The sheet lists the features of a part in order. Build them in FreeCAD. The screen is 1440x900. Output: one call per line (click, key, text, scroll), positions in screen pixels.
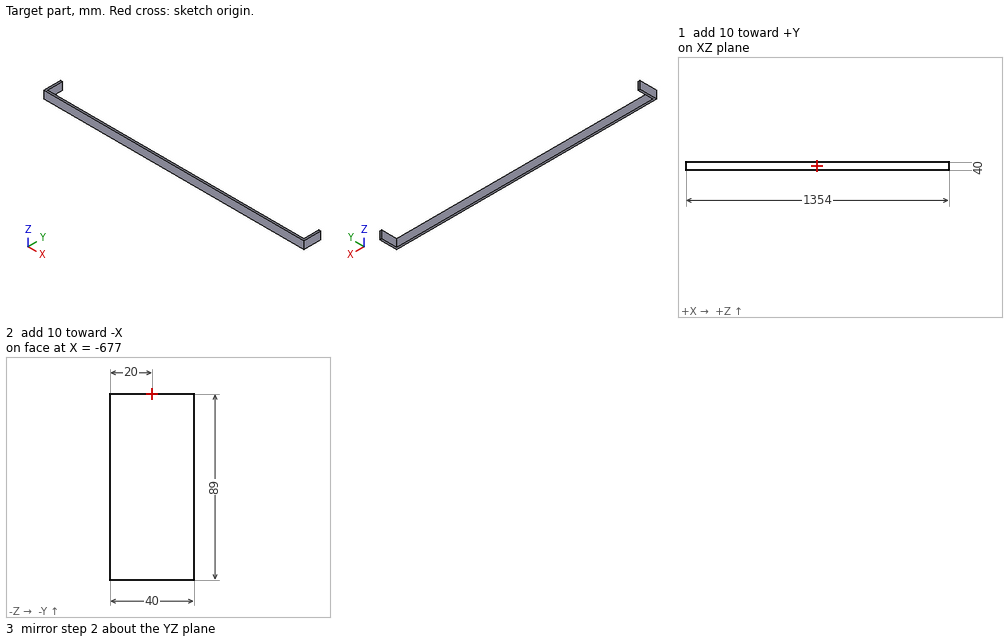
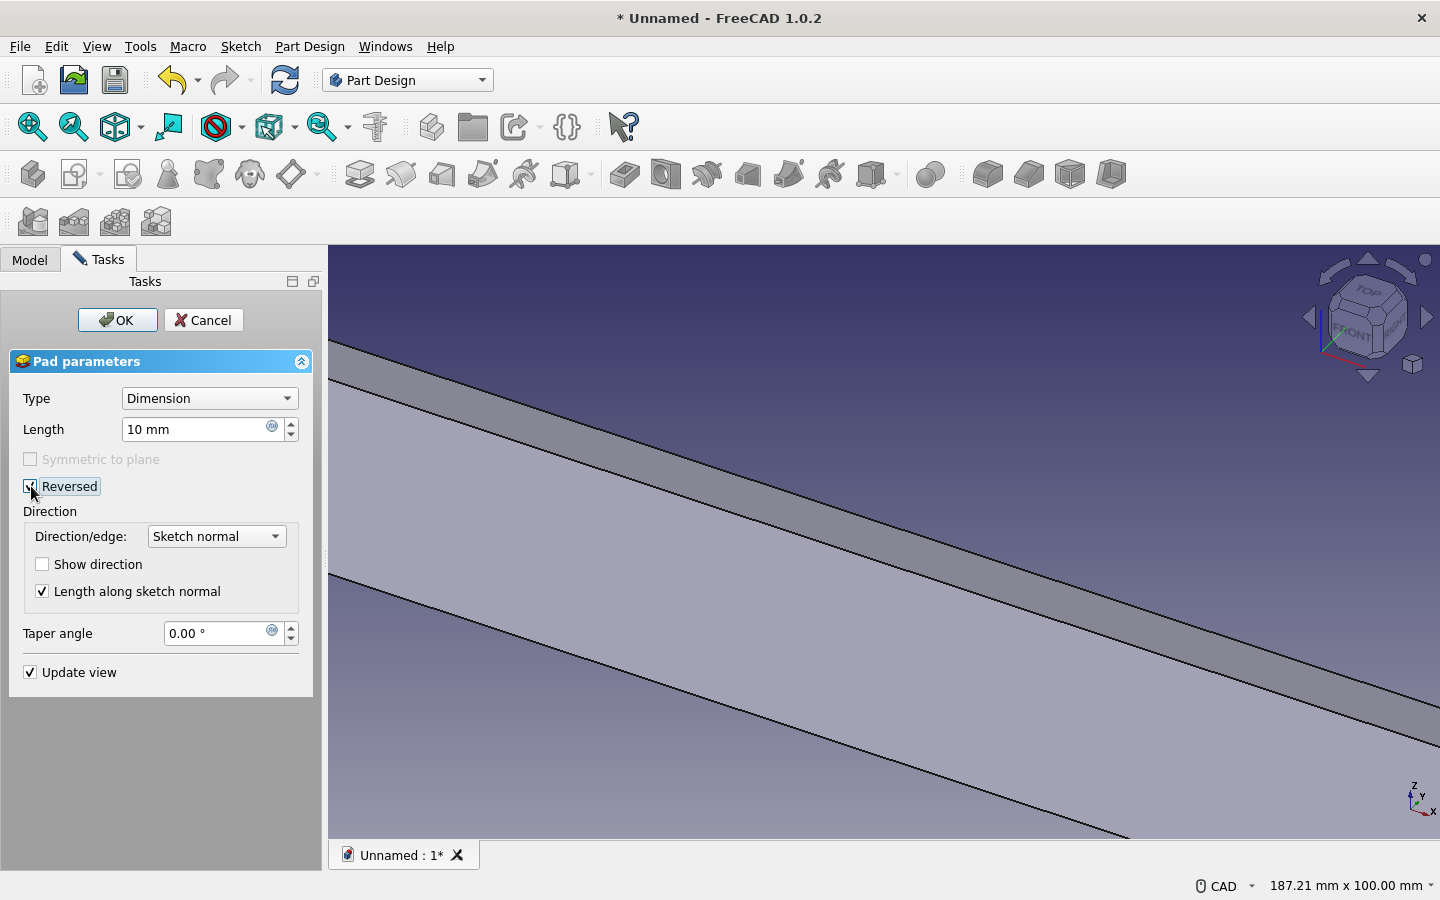
click(118, 320)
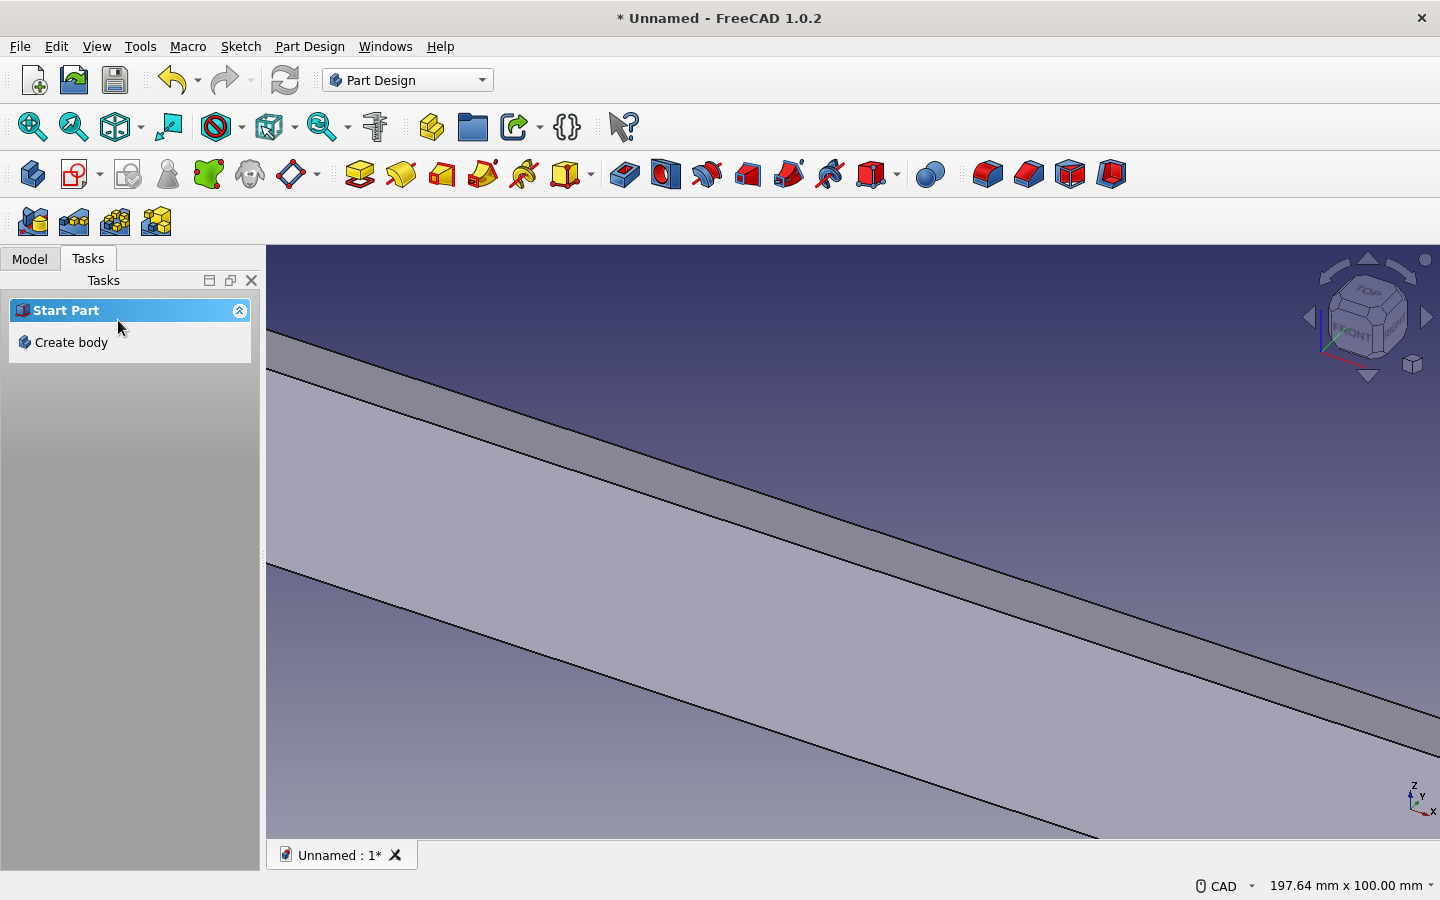
key(v)
key(f)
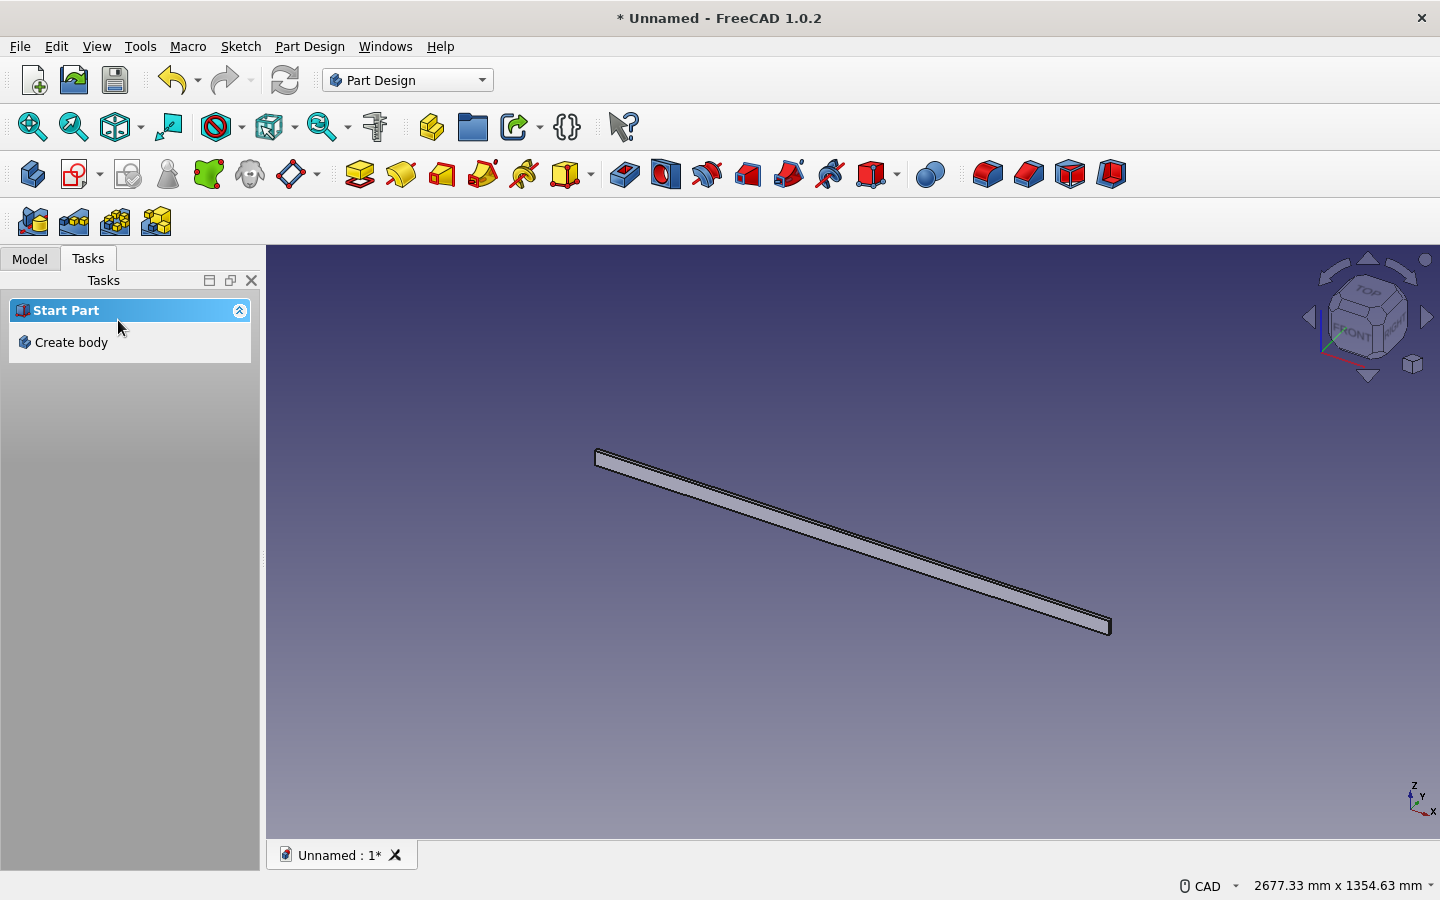
key(6)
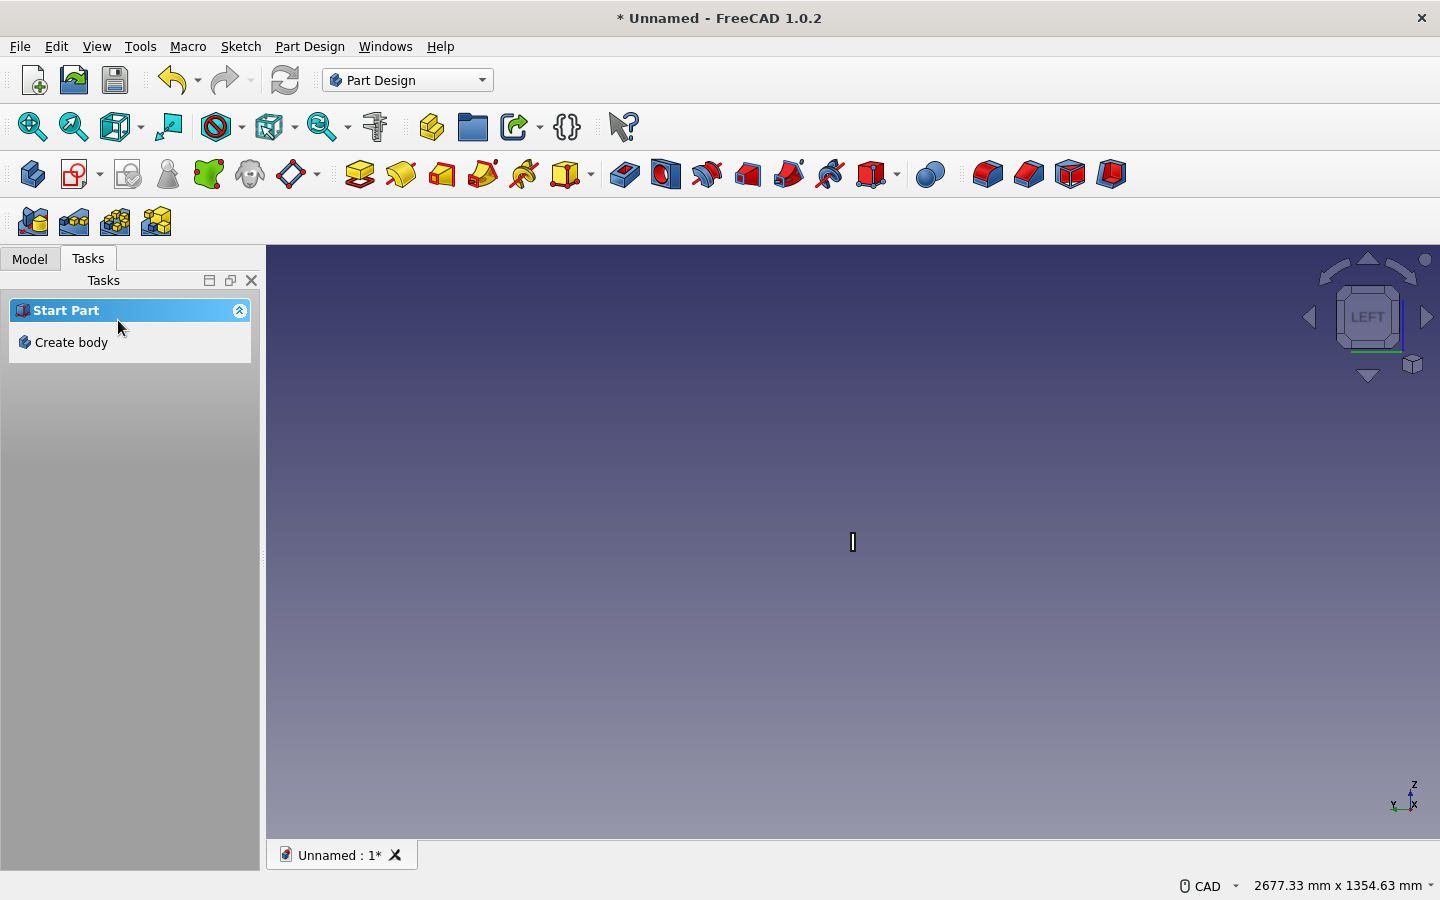
click(33, 128)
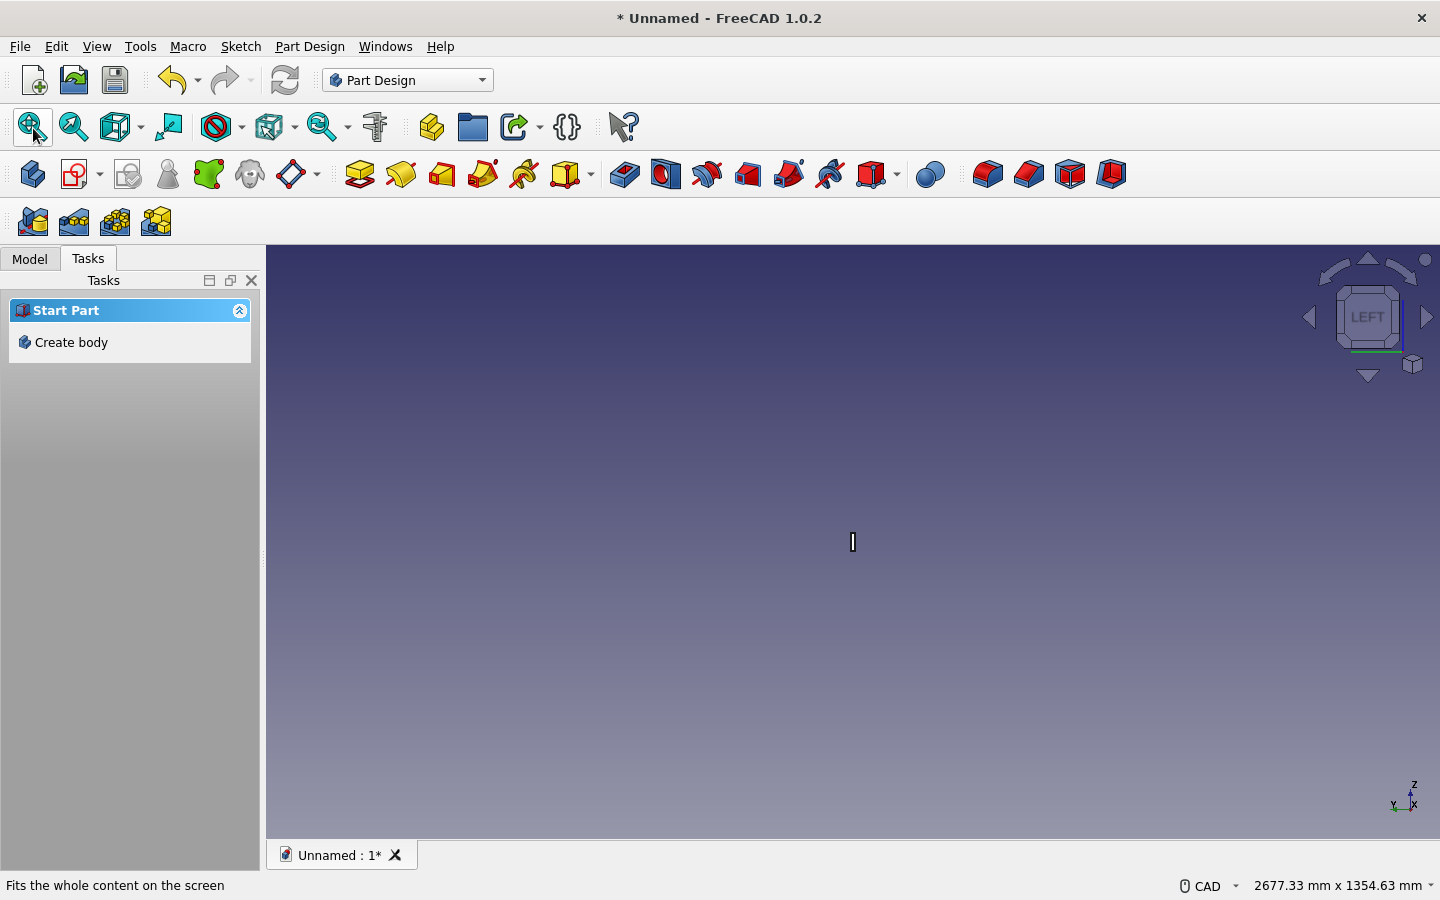
scroll(853, 536, up, 9)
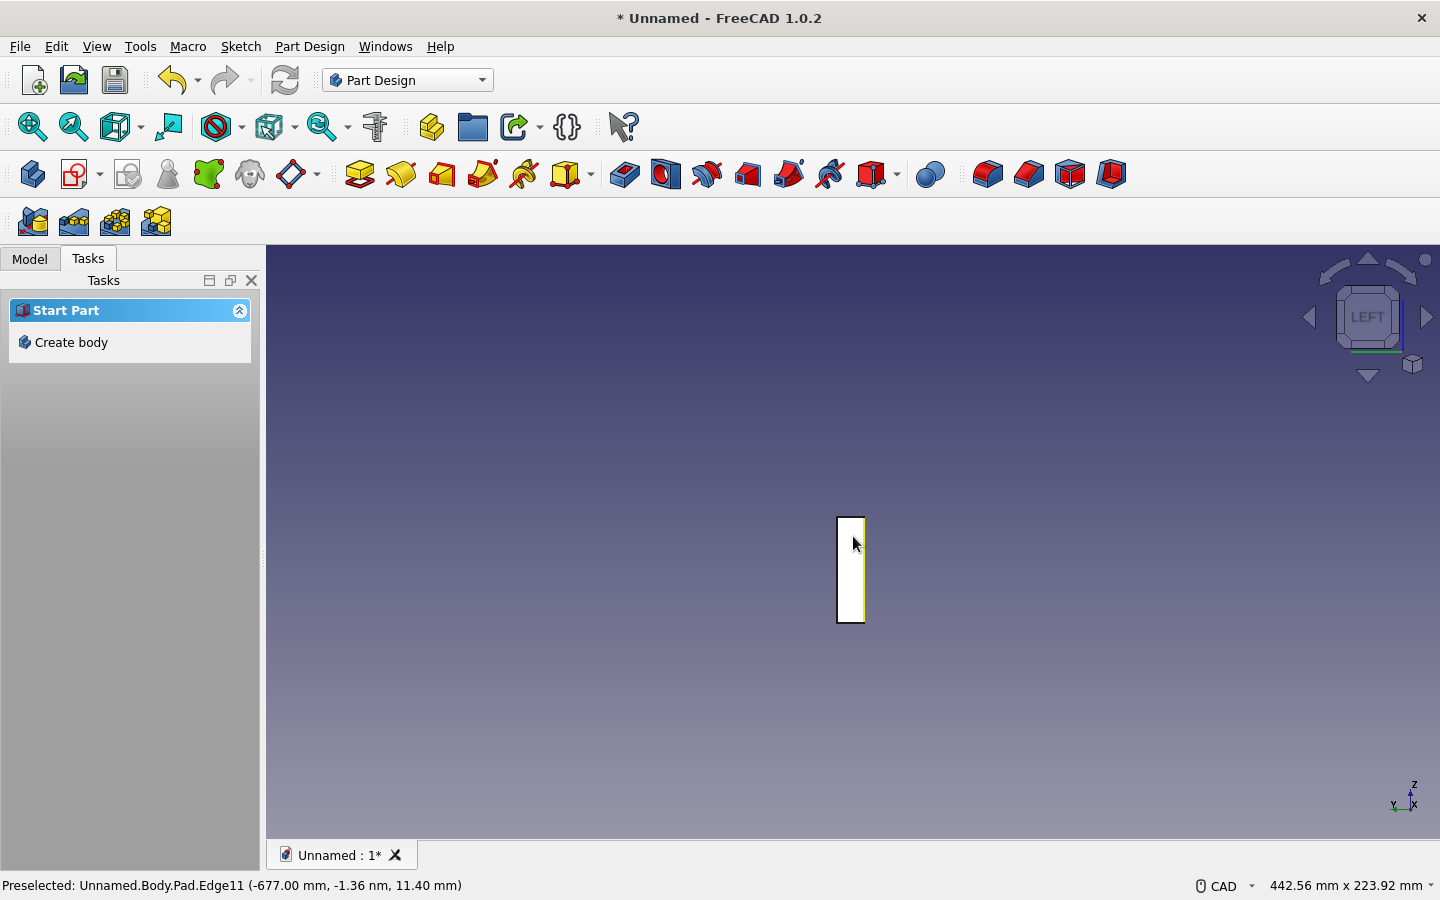
click(850, 539)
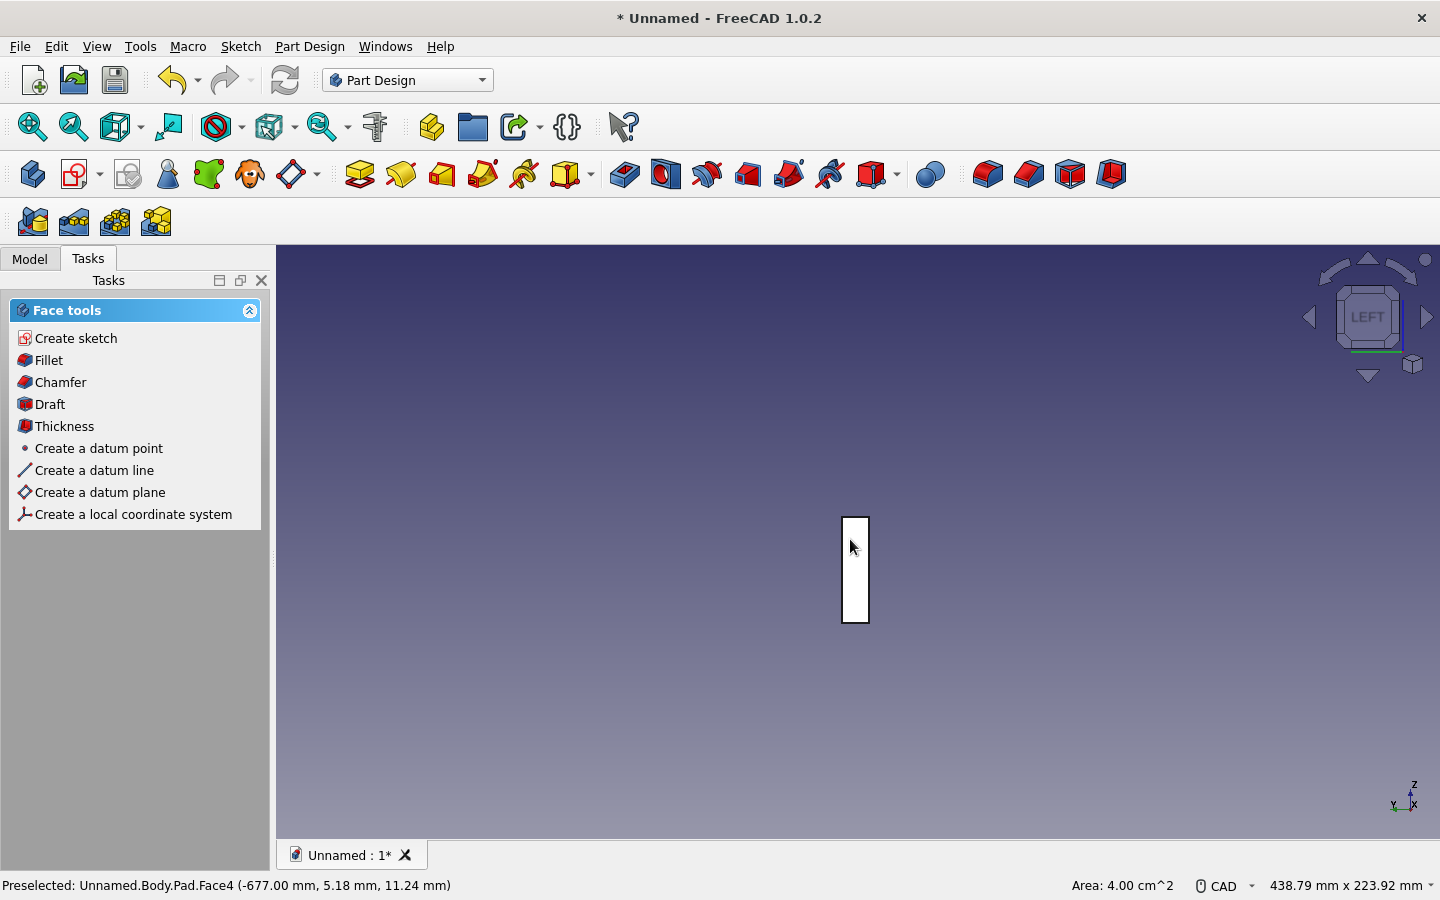
click(74, 174)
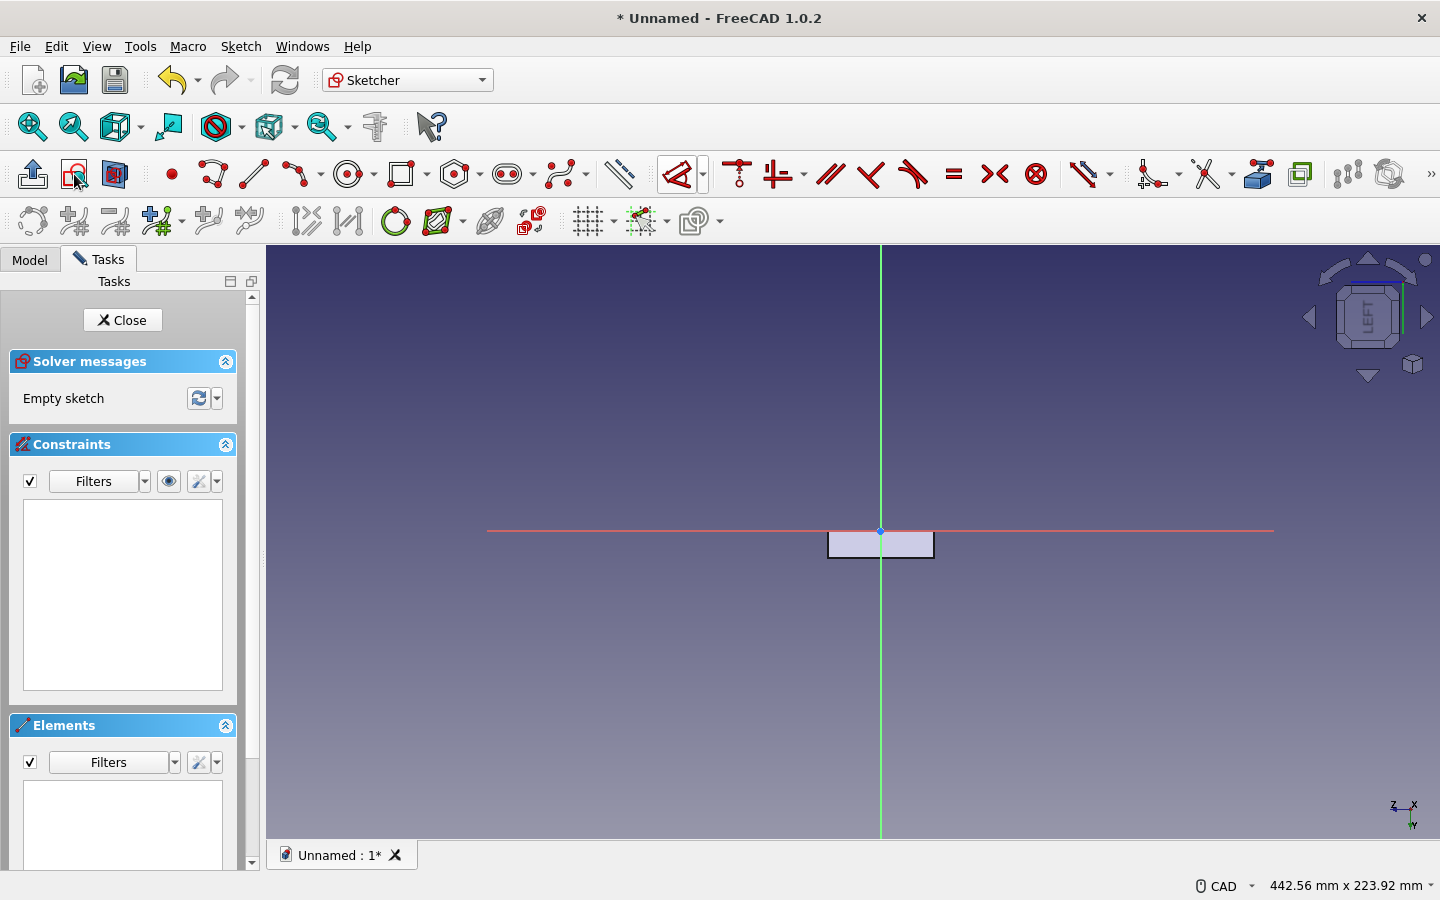
scroll(1077, 811, up, 2)